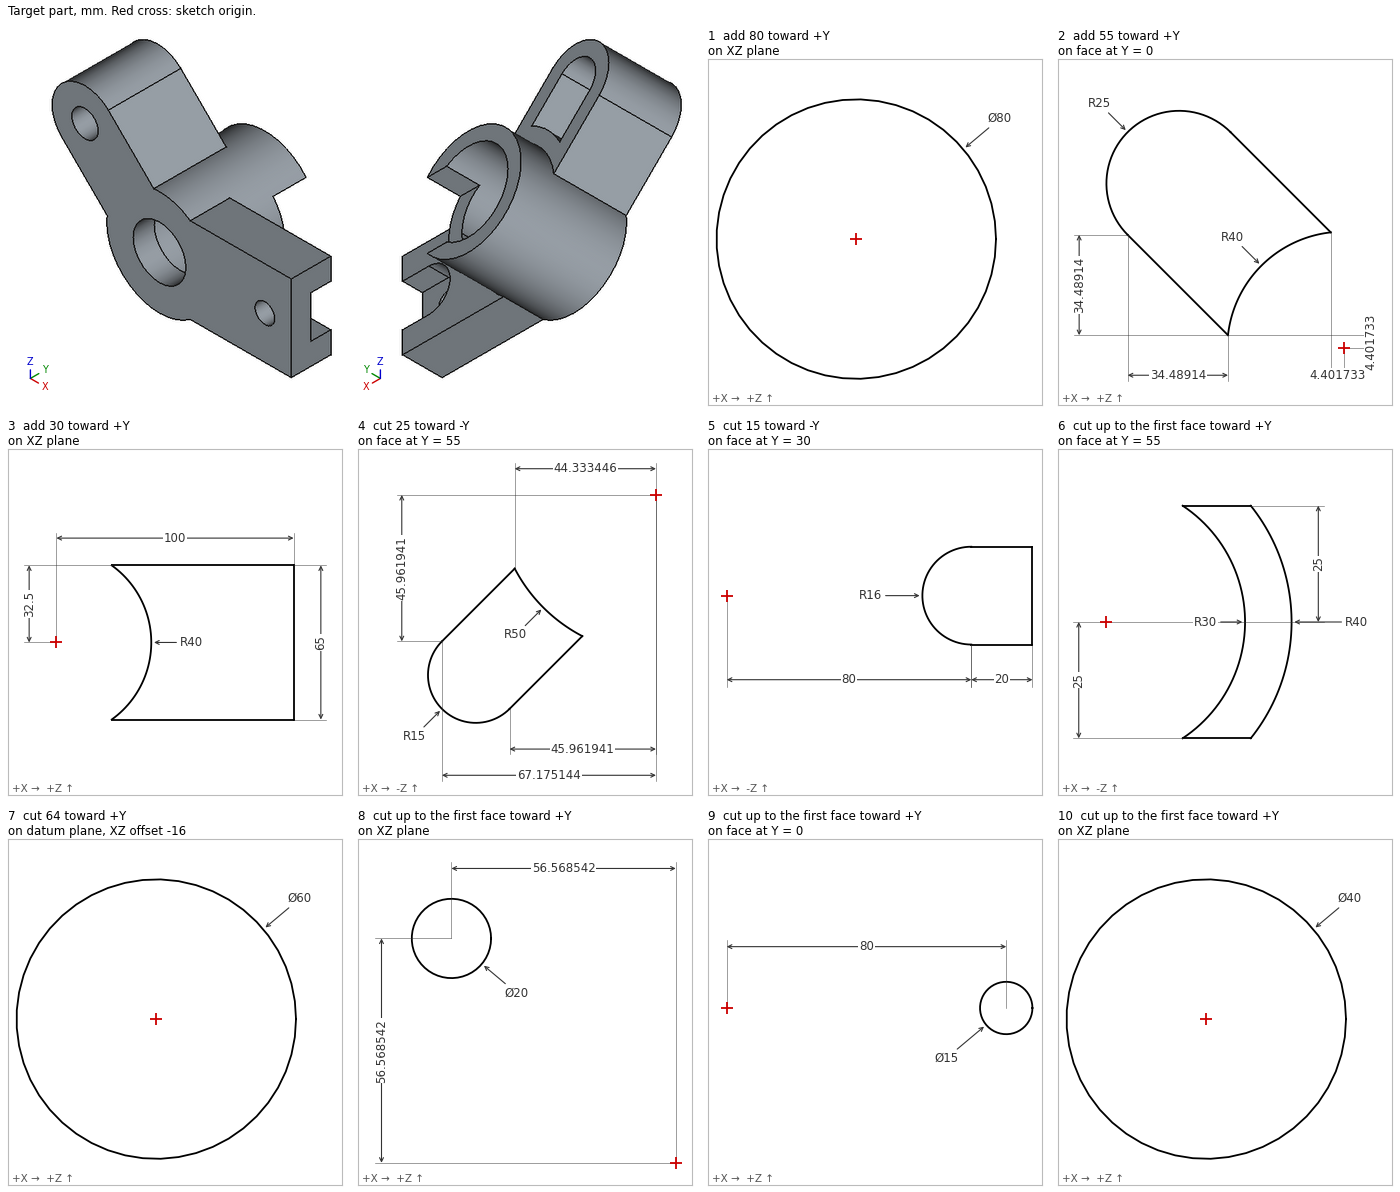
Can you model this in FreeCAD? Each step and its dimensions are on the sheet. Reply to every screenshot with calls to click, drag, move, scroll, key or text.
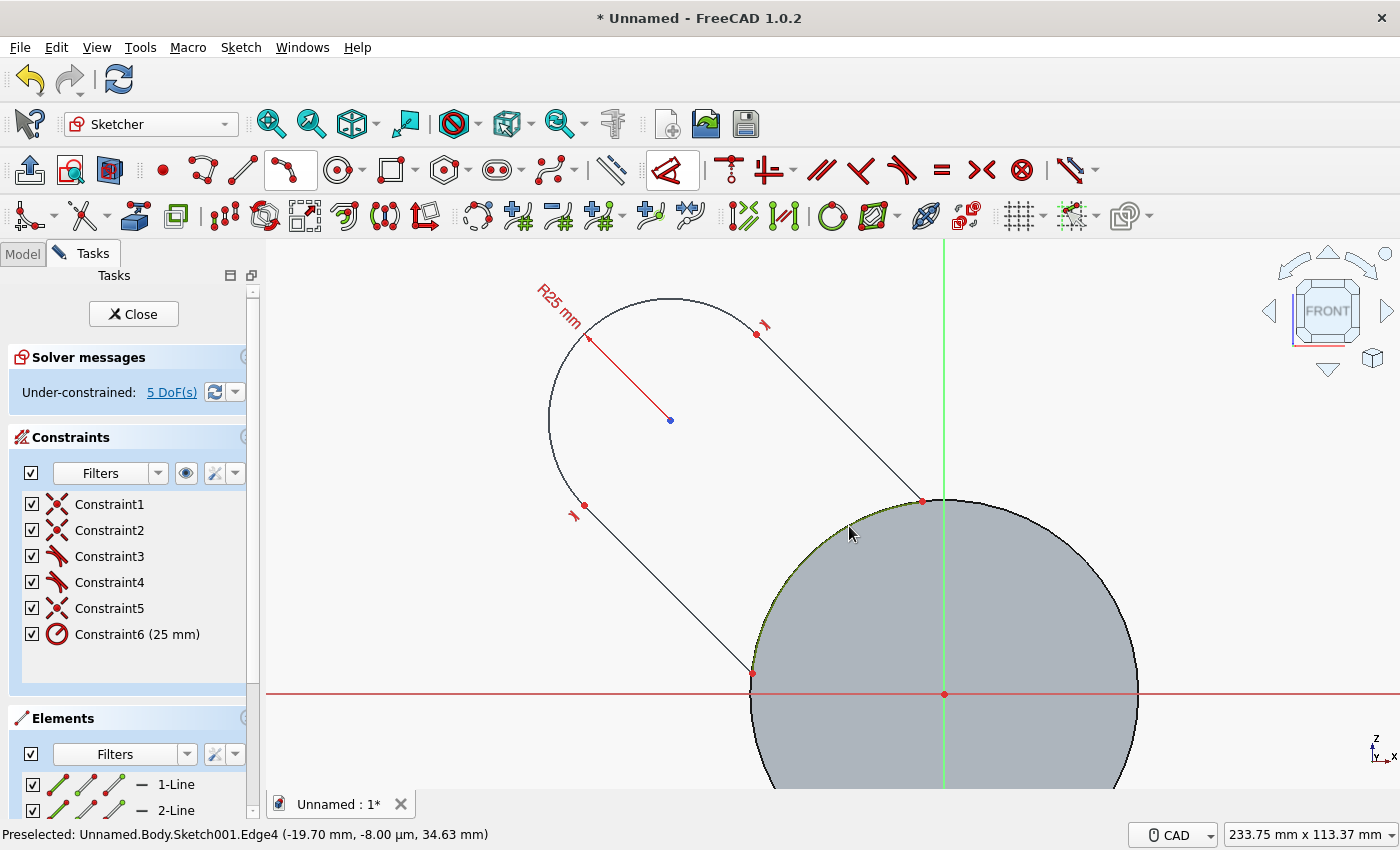
key(k)
key(r)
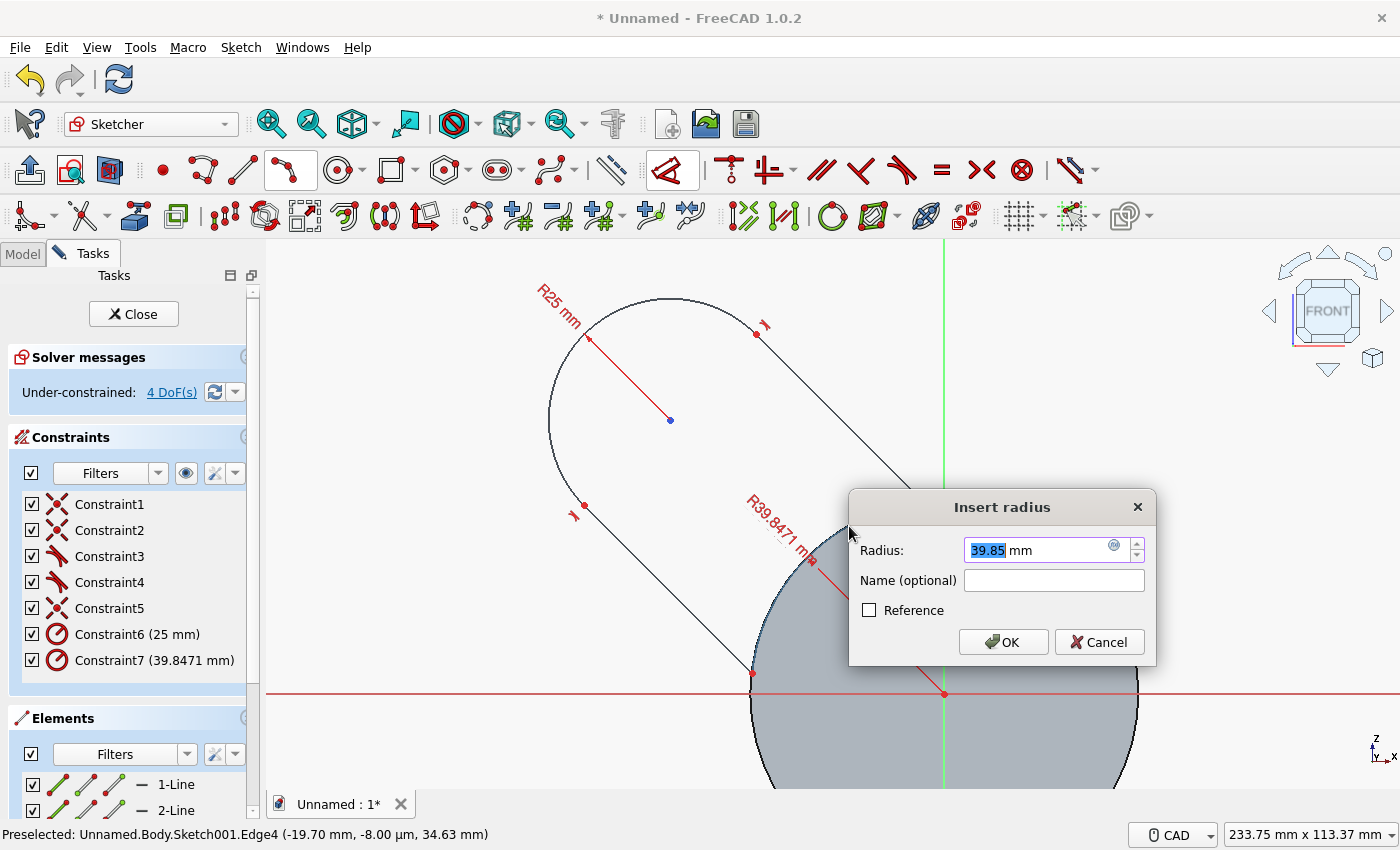
text(40)
key(Return)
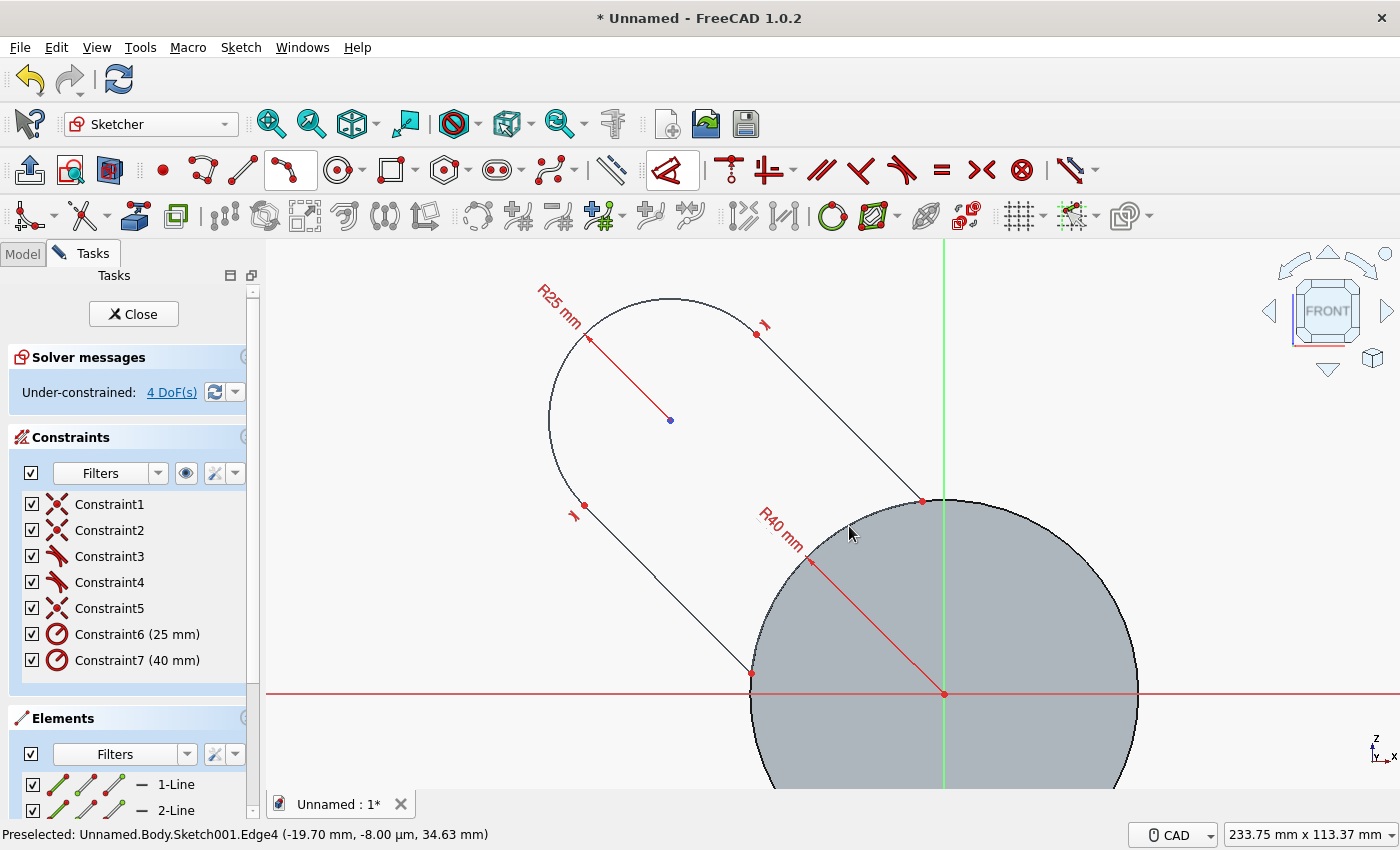
scroll(751, 674, up, 4)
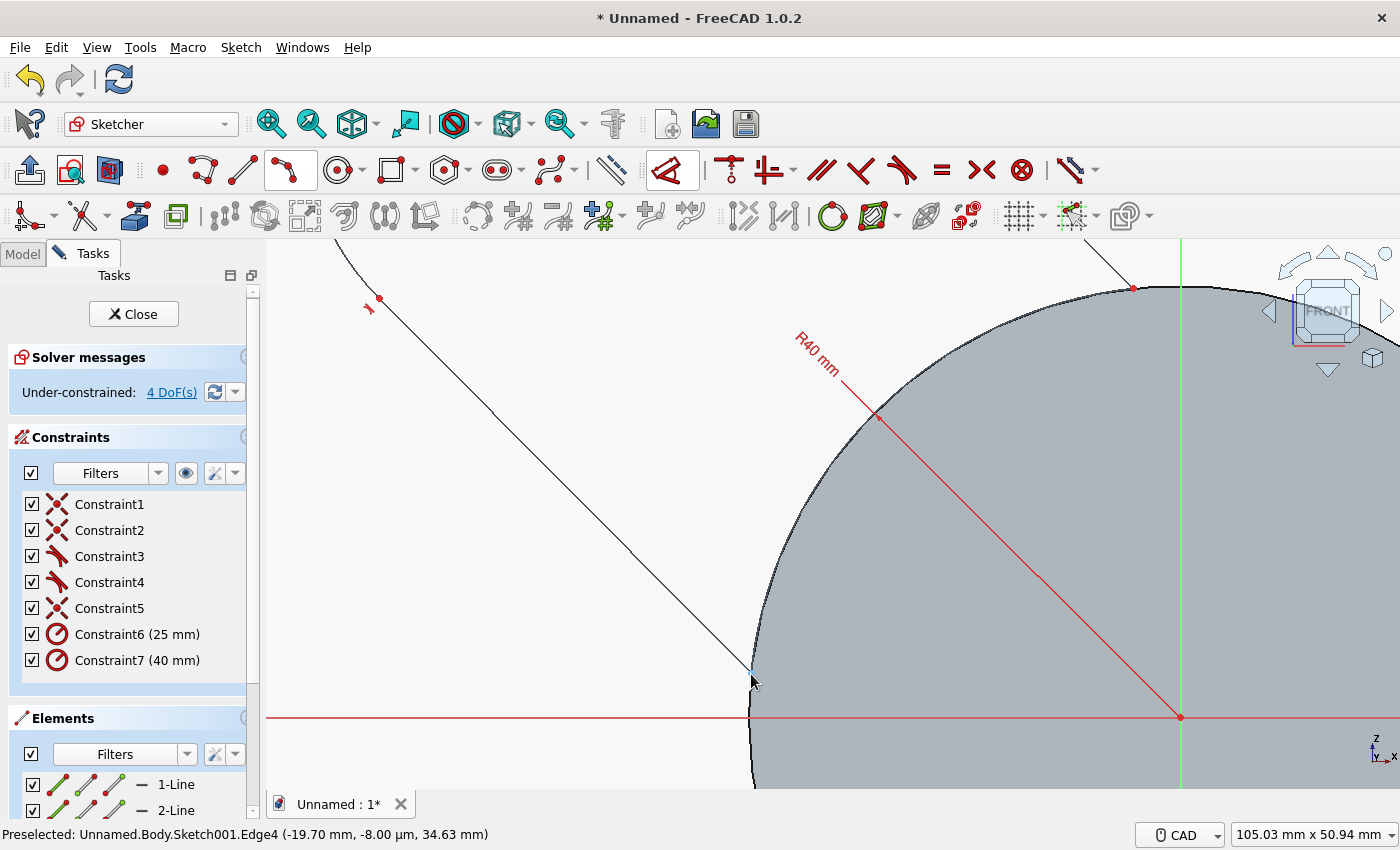
click(751, 673)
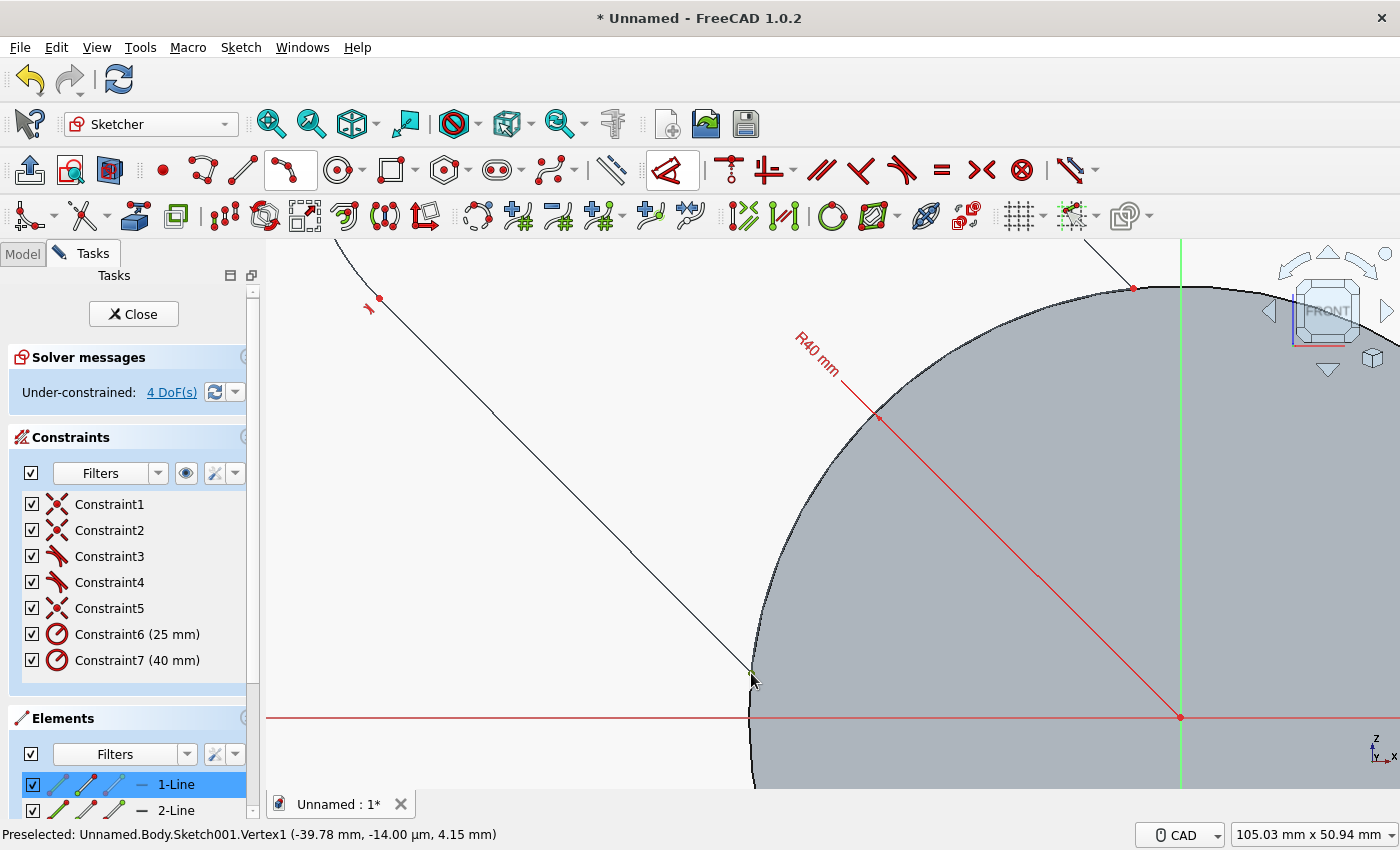
click(694, 170)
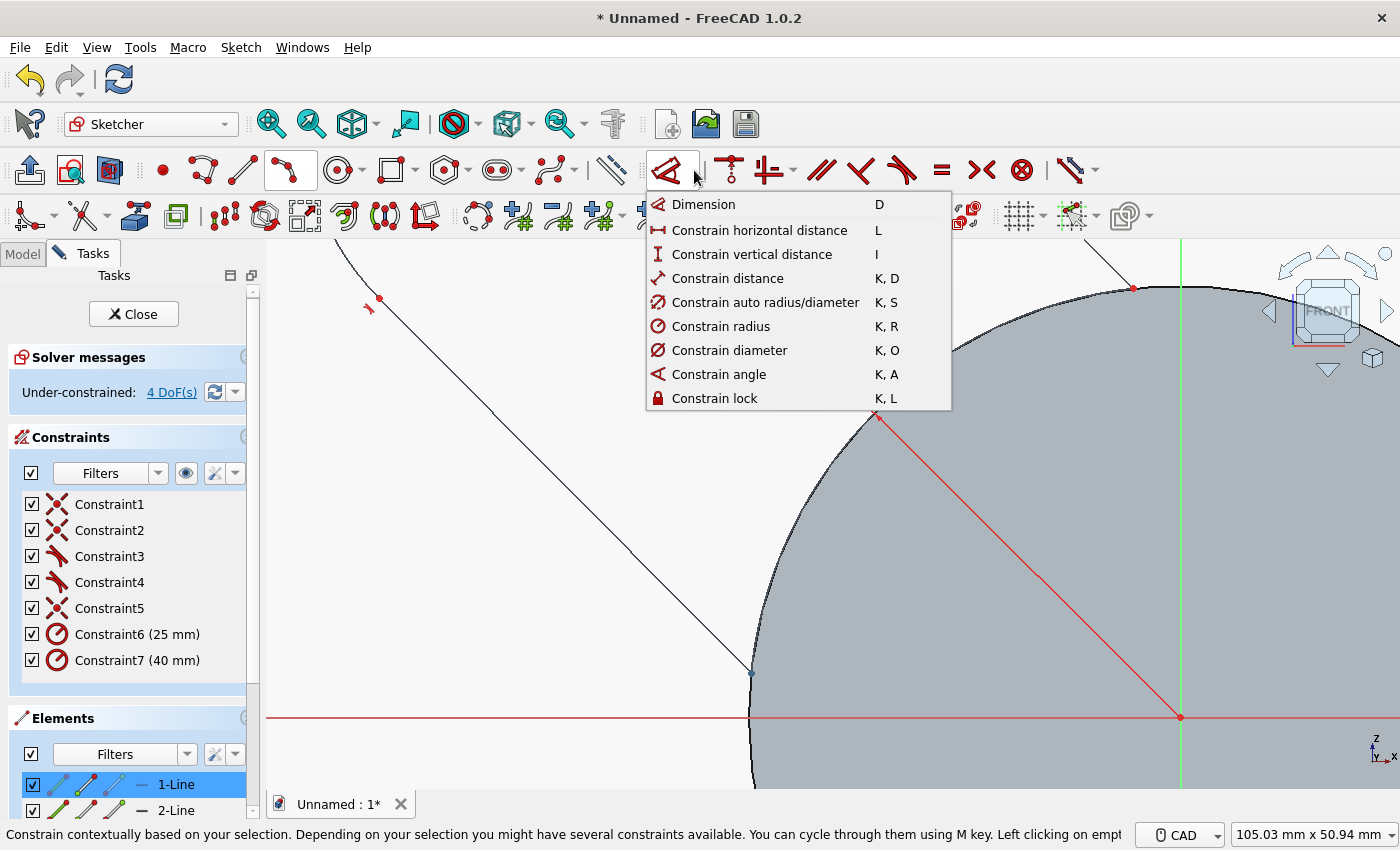
click(799, 254)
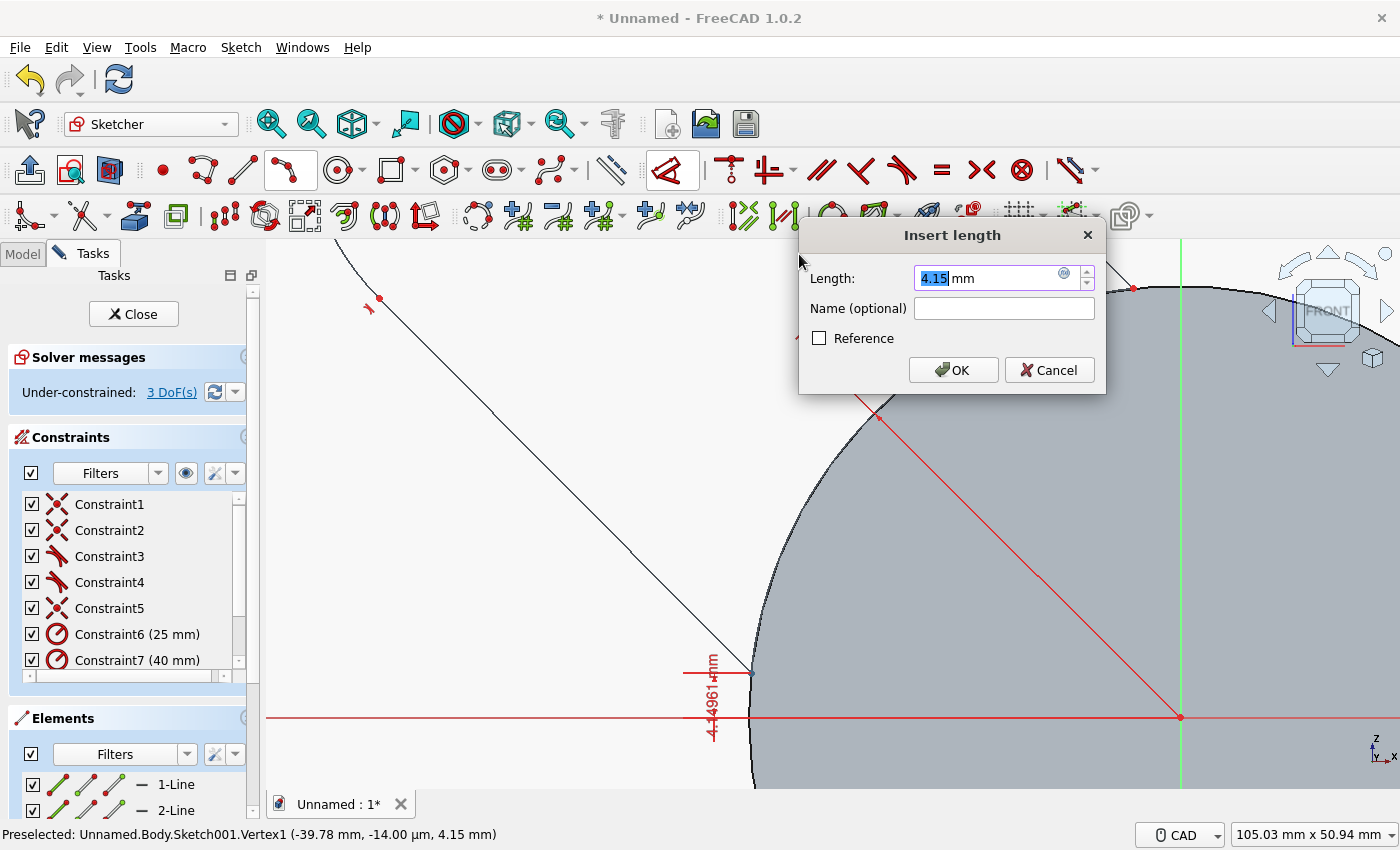
text(4.401733)
key(Return)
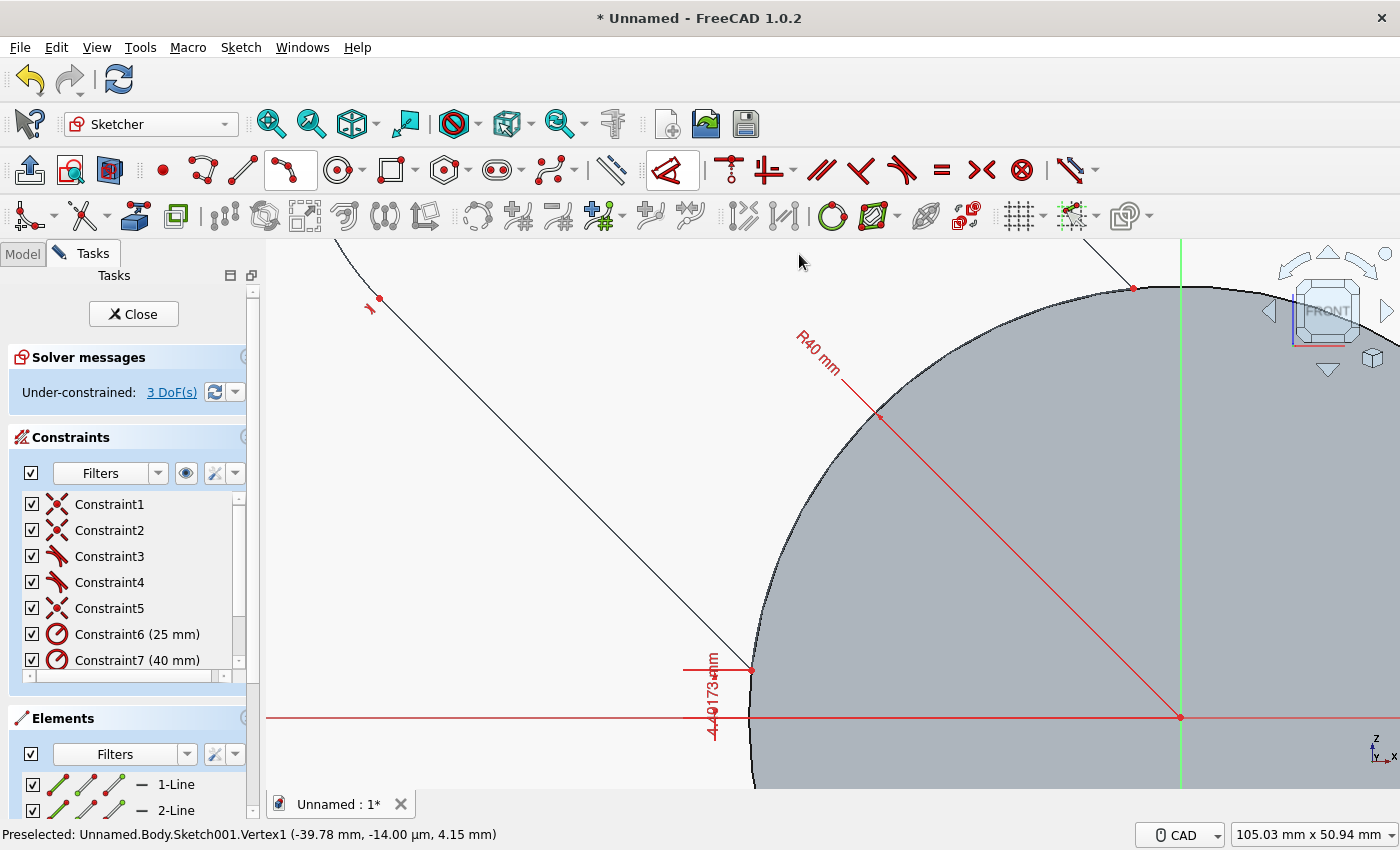
click(1133, 289)